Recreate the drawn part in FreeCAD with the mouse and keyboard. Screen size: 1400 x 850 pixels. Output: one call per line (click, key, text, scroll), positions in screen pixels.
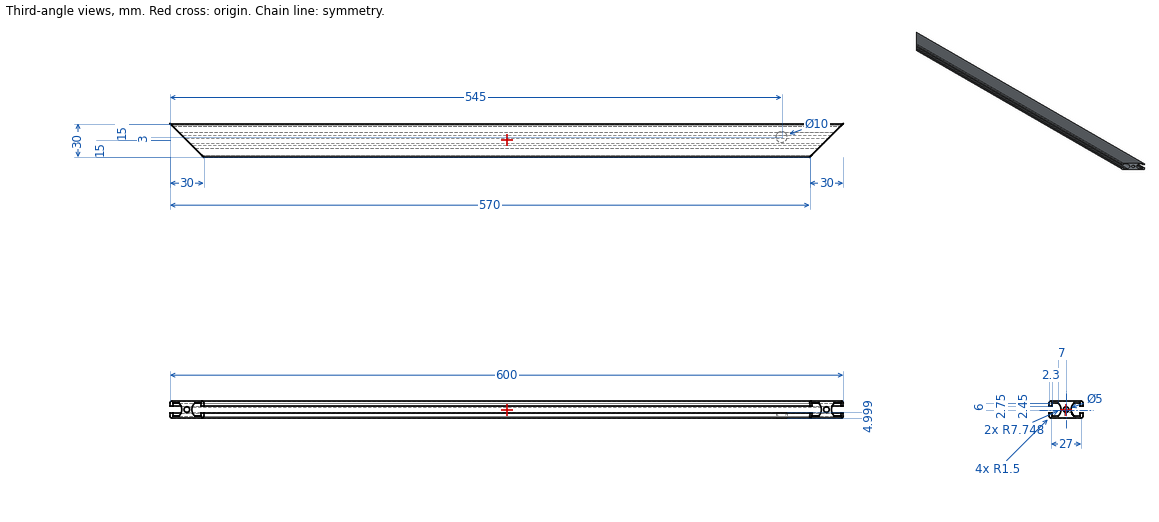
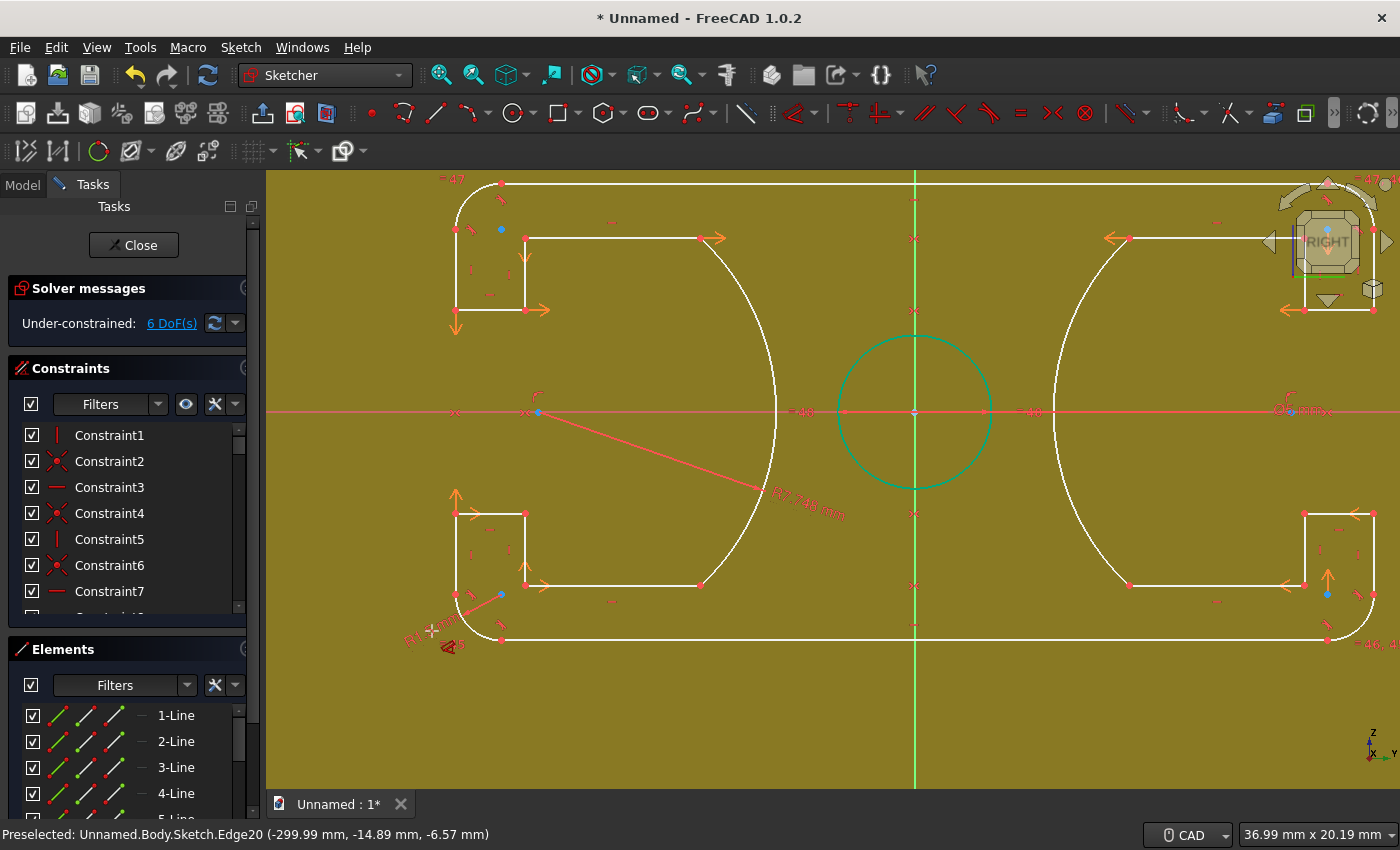
click(750, 640)
click(868, 674)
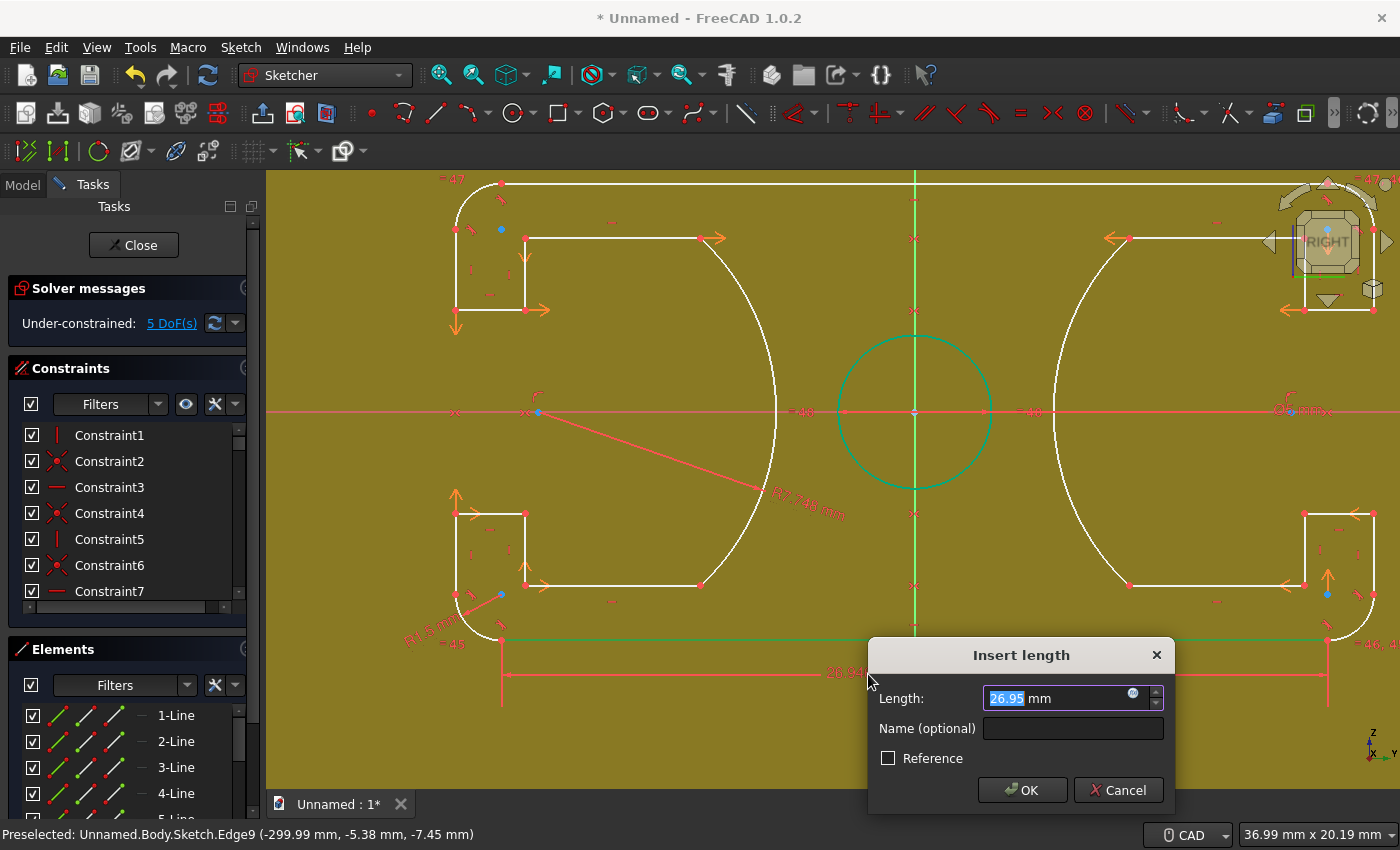
text(27)
key(Return)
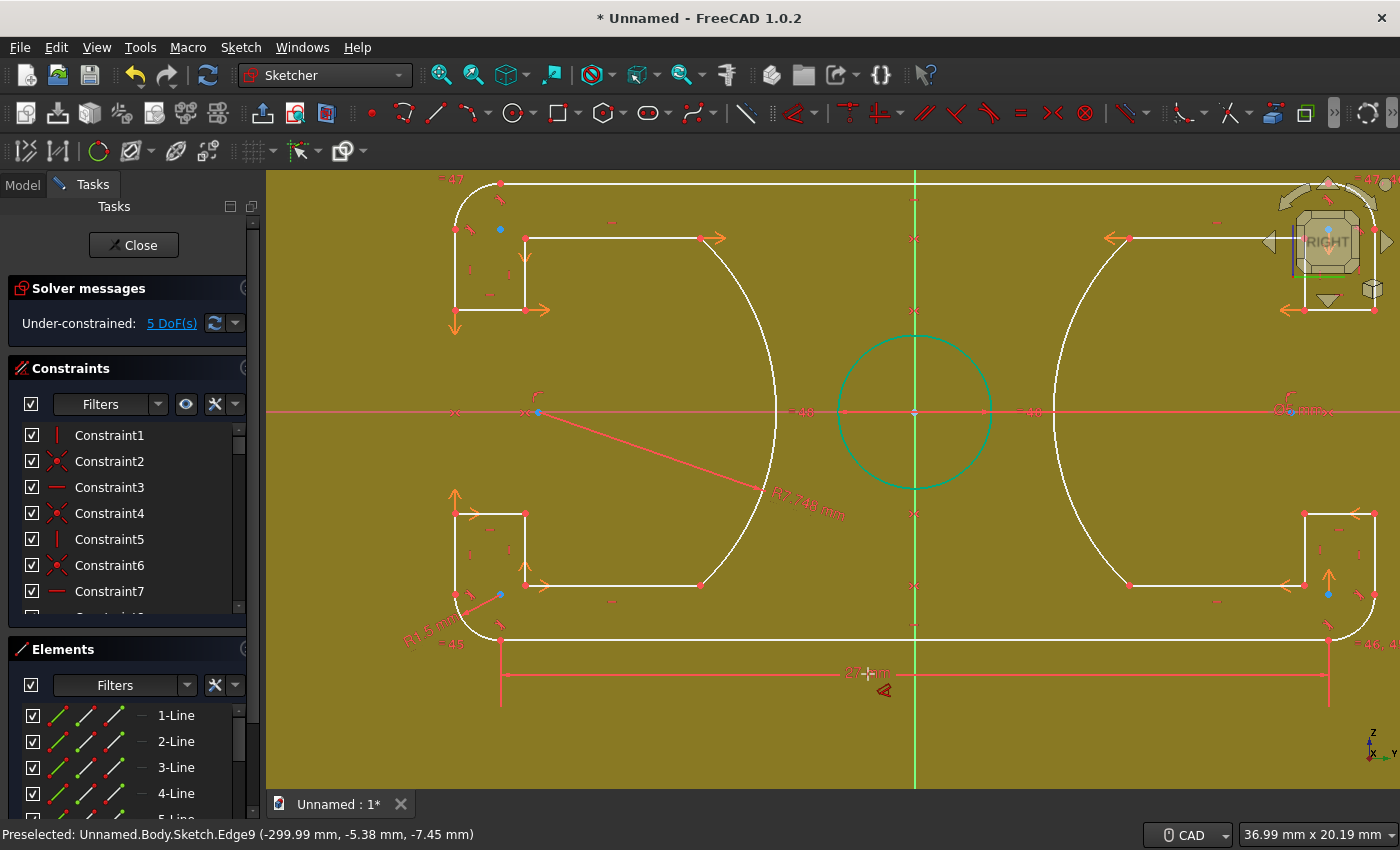
click(455, 230)
click(421, 321)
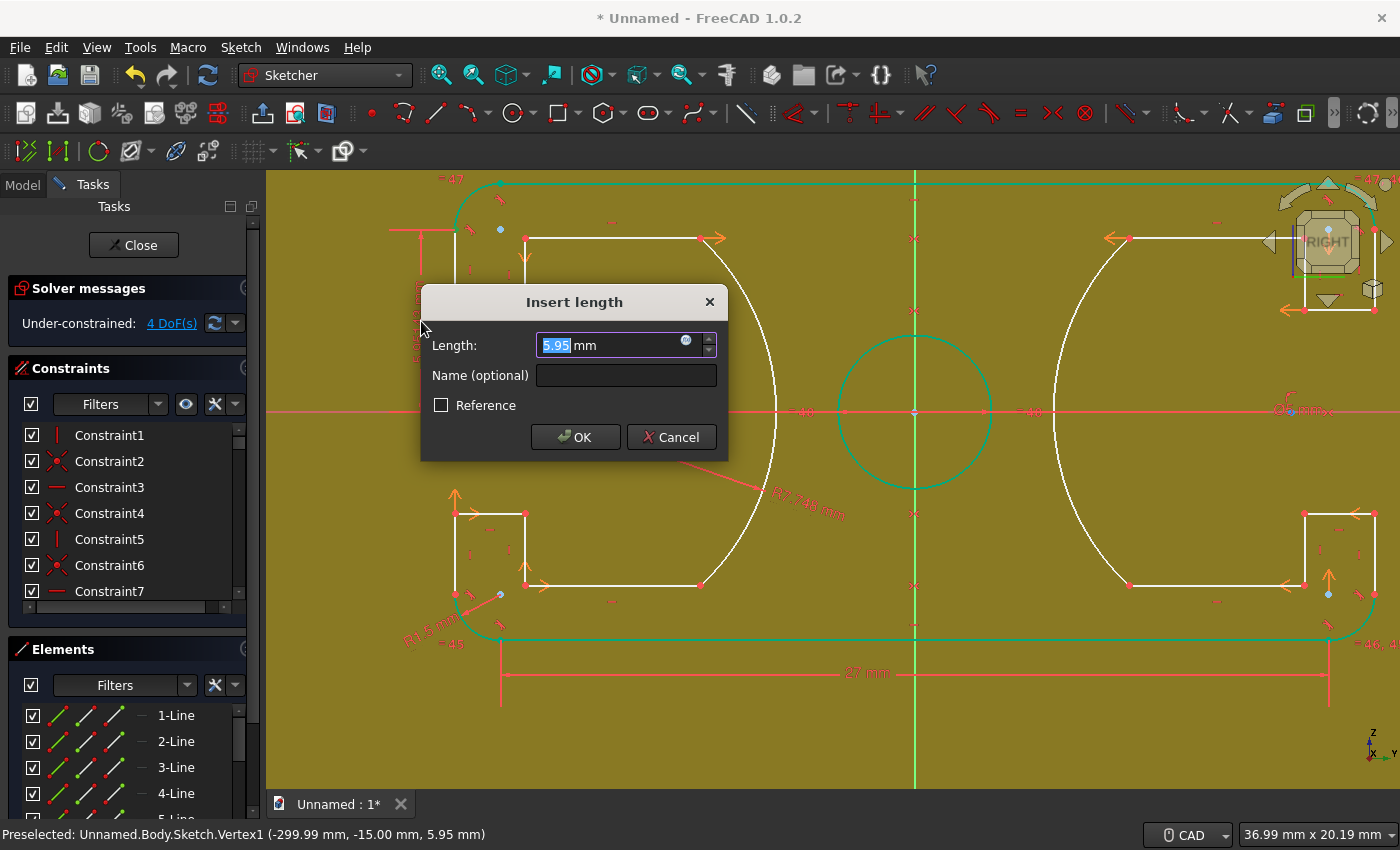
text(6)
key(Return)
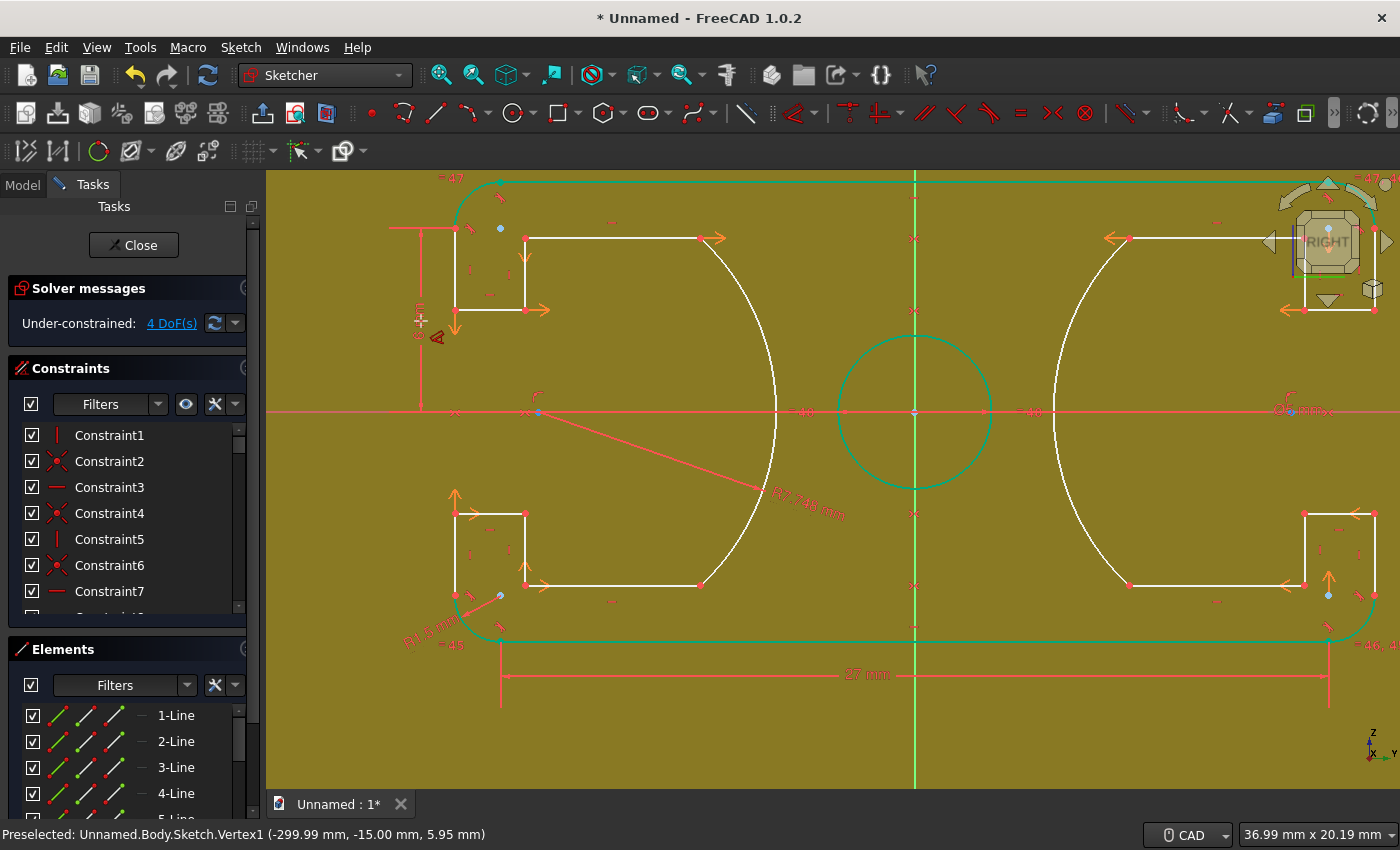
click(701, 238)
click(808, 204)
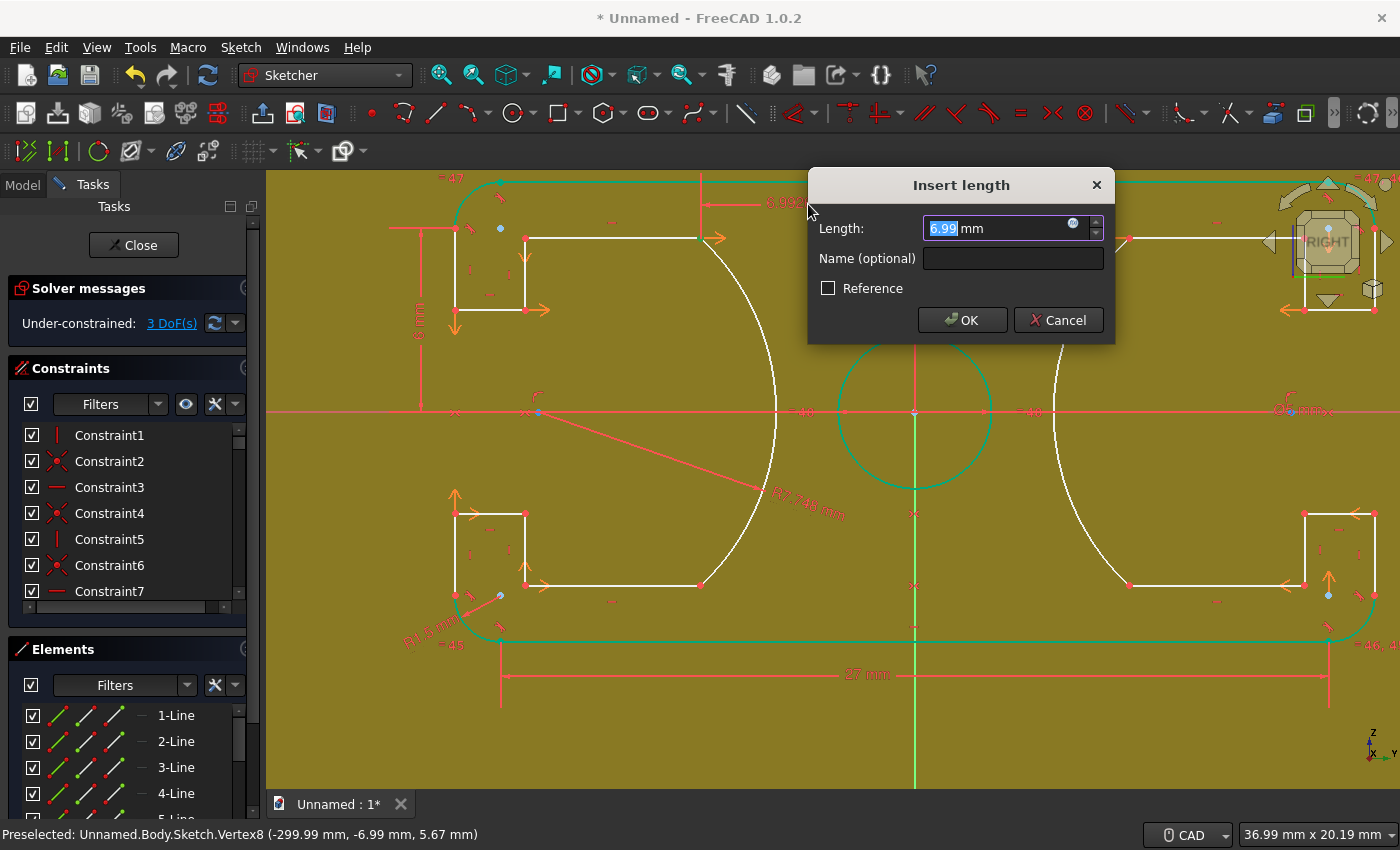
text(7)
key(Return)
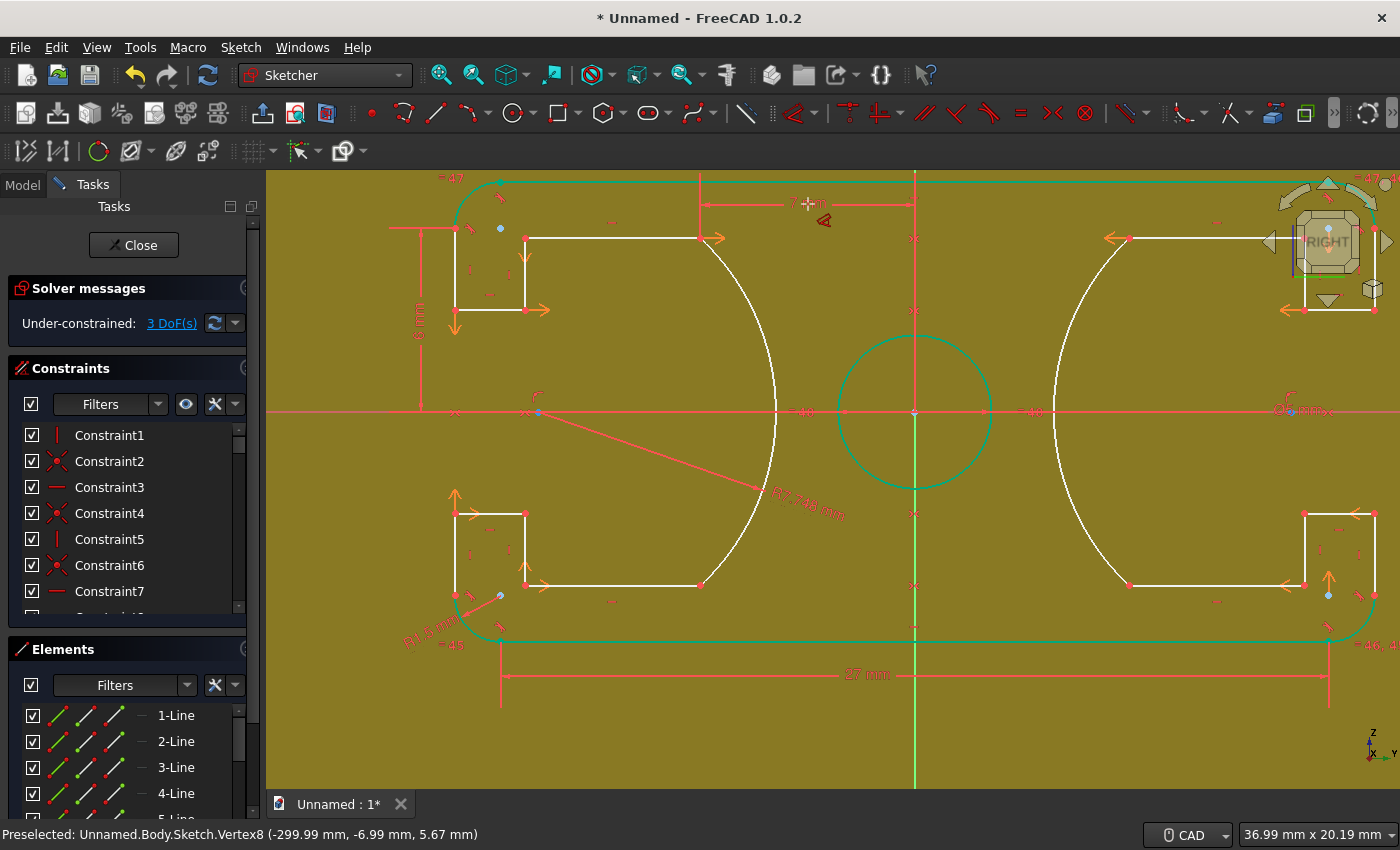
click(476, 310)
click(490, 276)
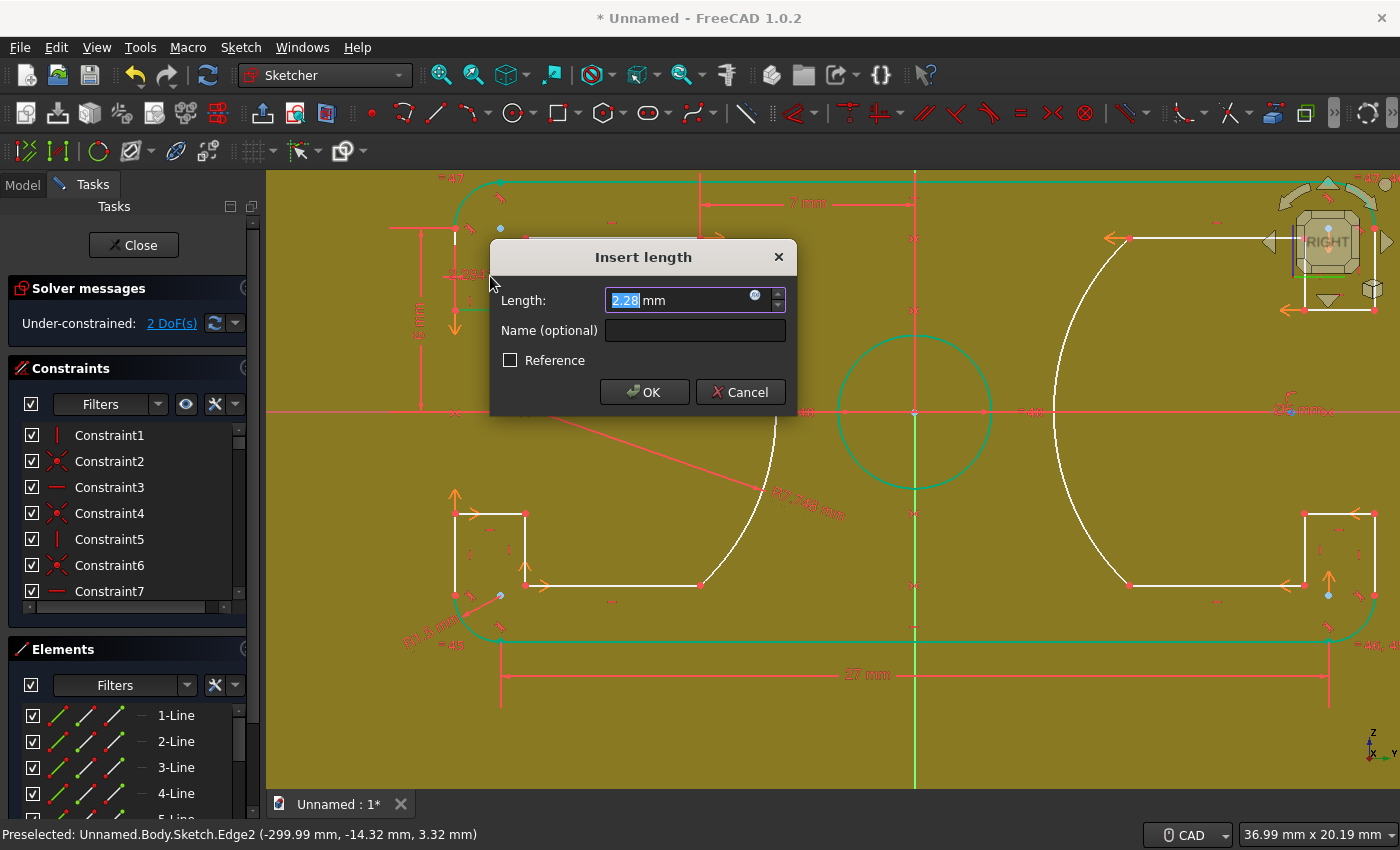
text(2.3)
key(Return)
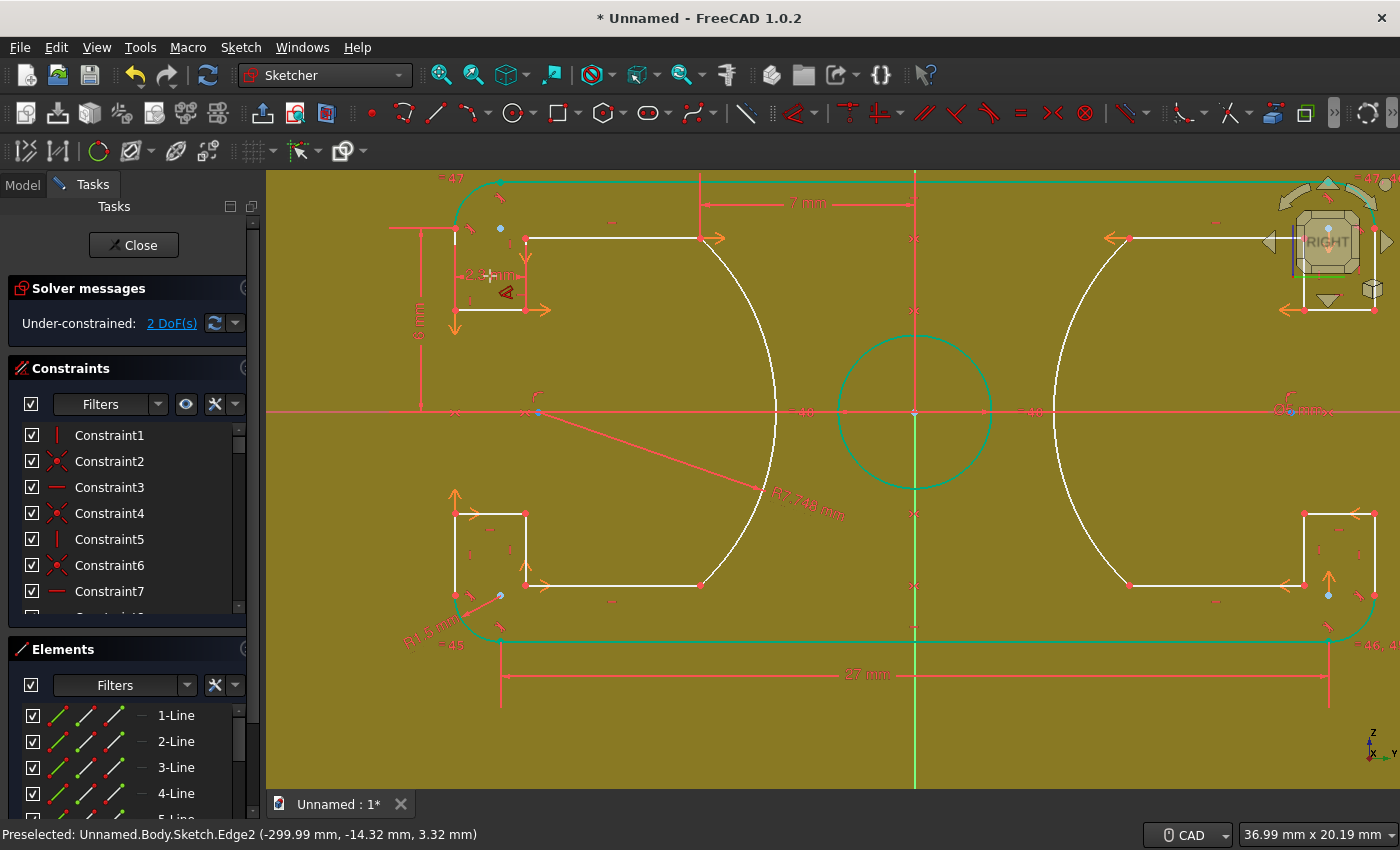
click(455, 253)
click(421, 250)